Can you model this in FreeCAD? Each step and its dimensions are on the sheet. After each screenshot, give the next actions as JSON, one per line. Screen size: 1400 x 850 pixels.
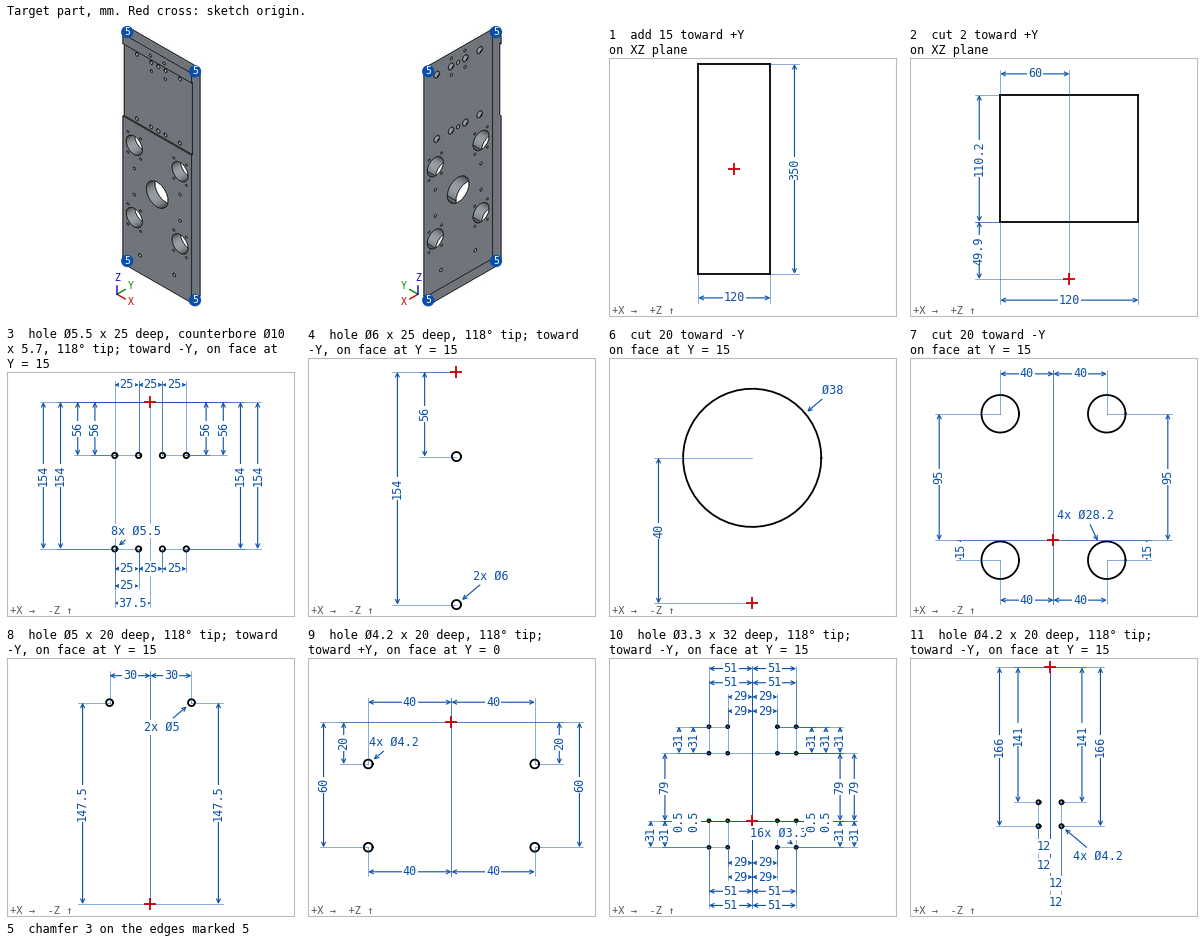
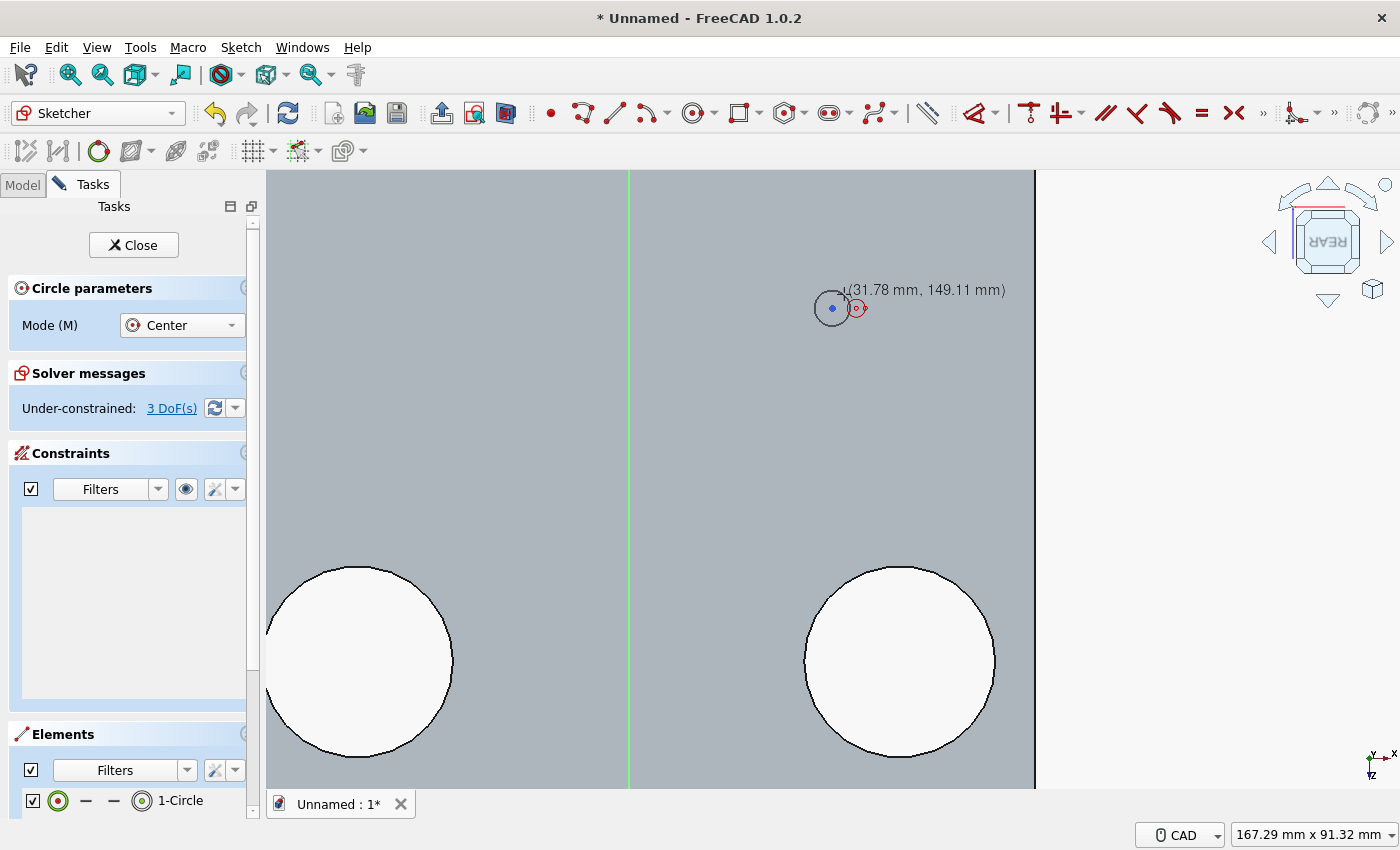
{"action": "scroll", "coordinate": [425, 306], "scroll_direction": "up", "scroll_amount": 2}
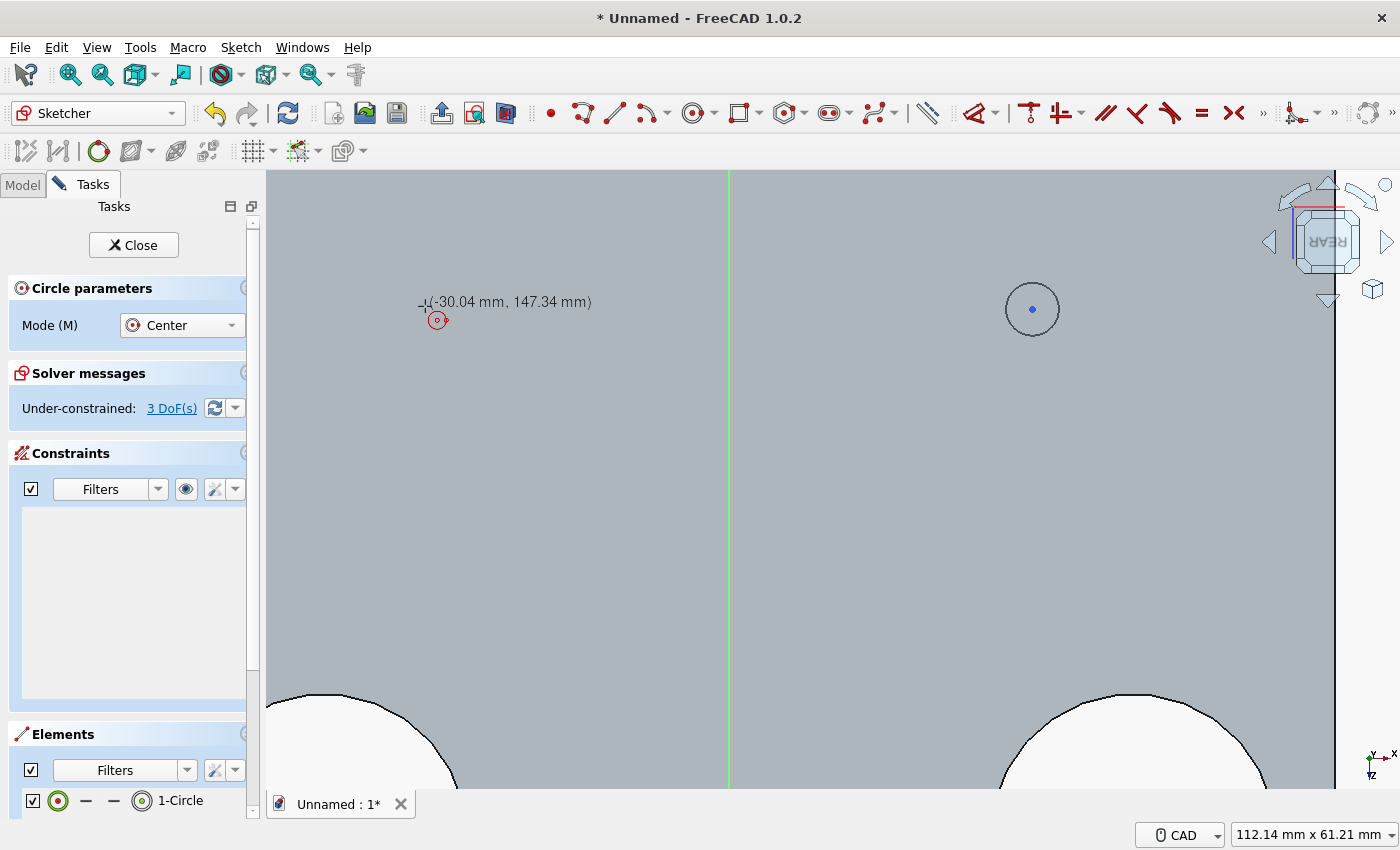
{"action": "scroll", "coordinate": [776, 296], "scroll_direction": "down", "scroll_amount": 7}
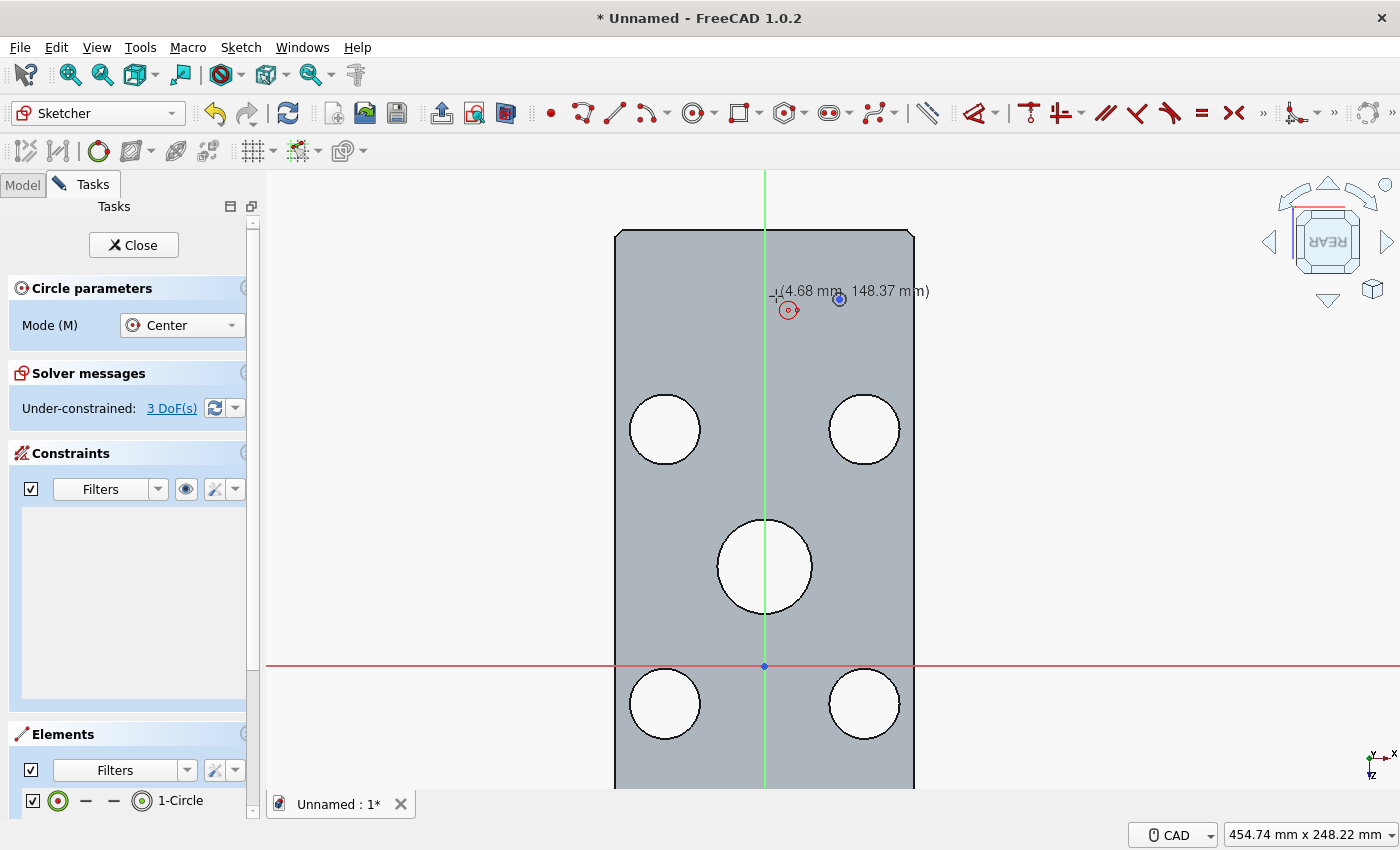
{"action": "left_click", "coordinate": [690, 299]}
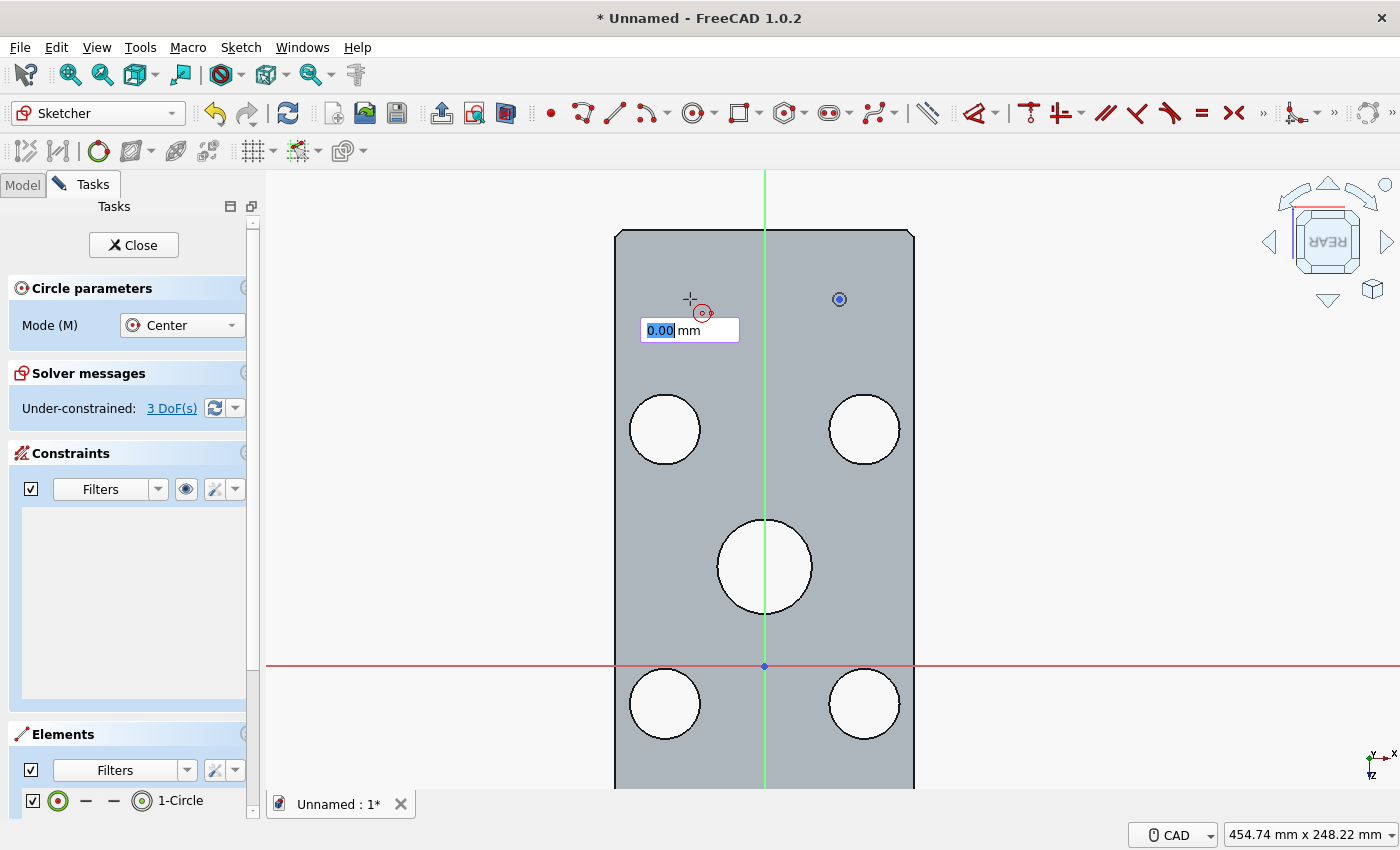
{"action": "scroll", "coordinate": [694, 294], "scroll_direction": "up", "scroll_amount": 5}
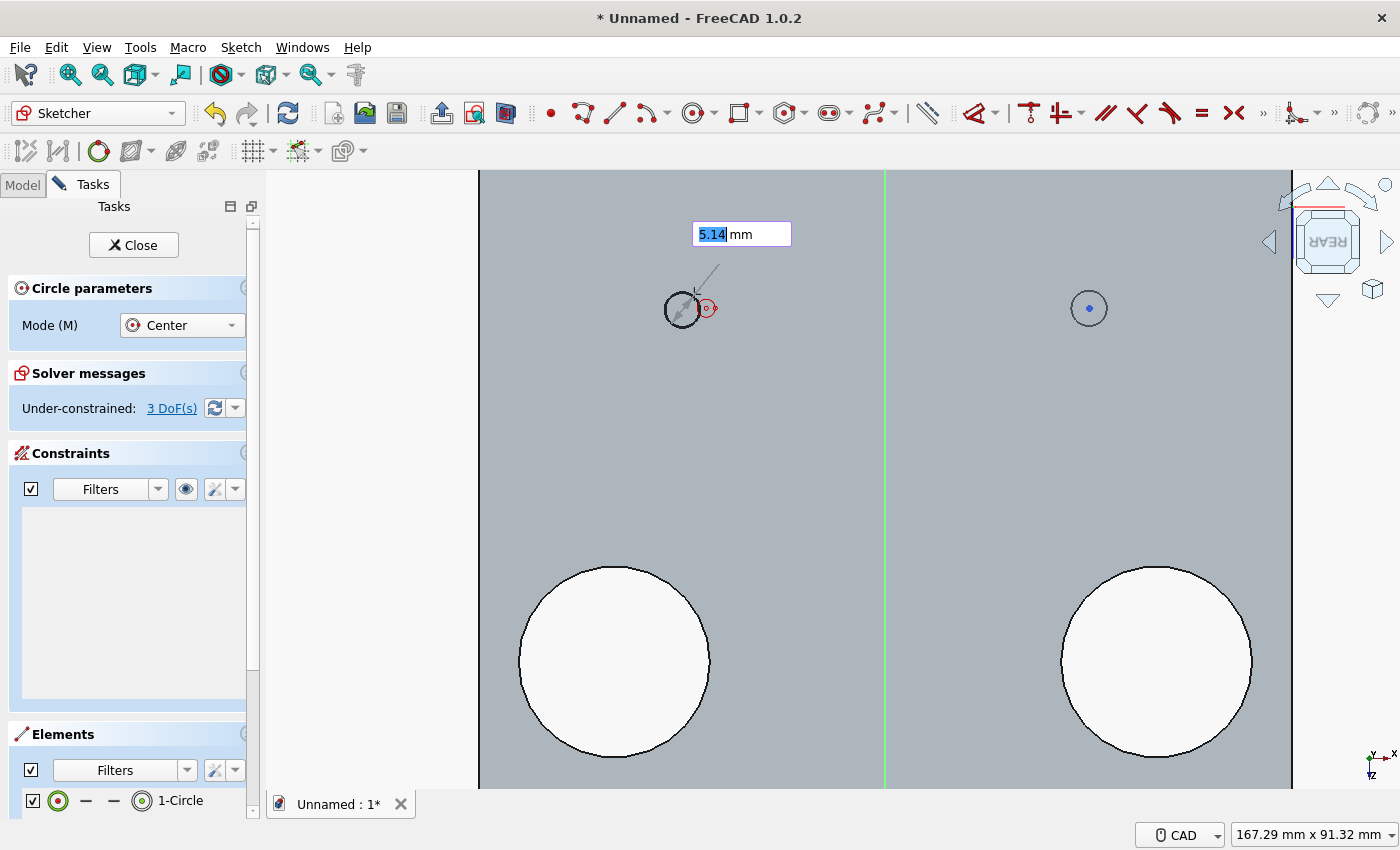
{"action": "left_click", "coordinate": [694, 294]}
{"action": "key", "text": "Escape"}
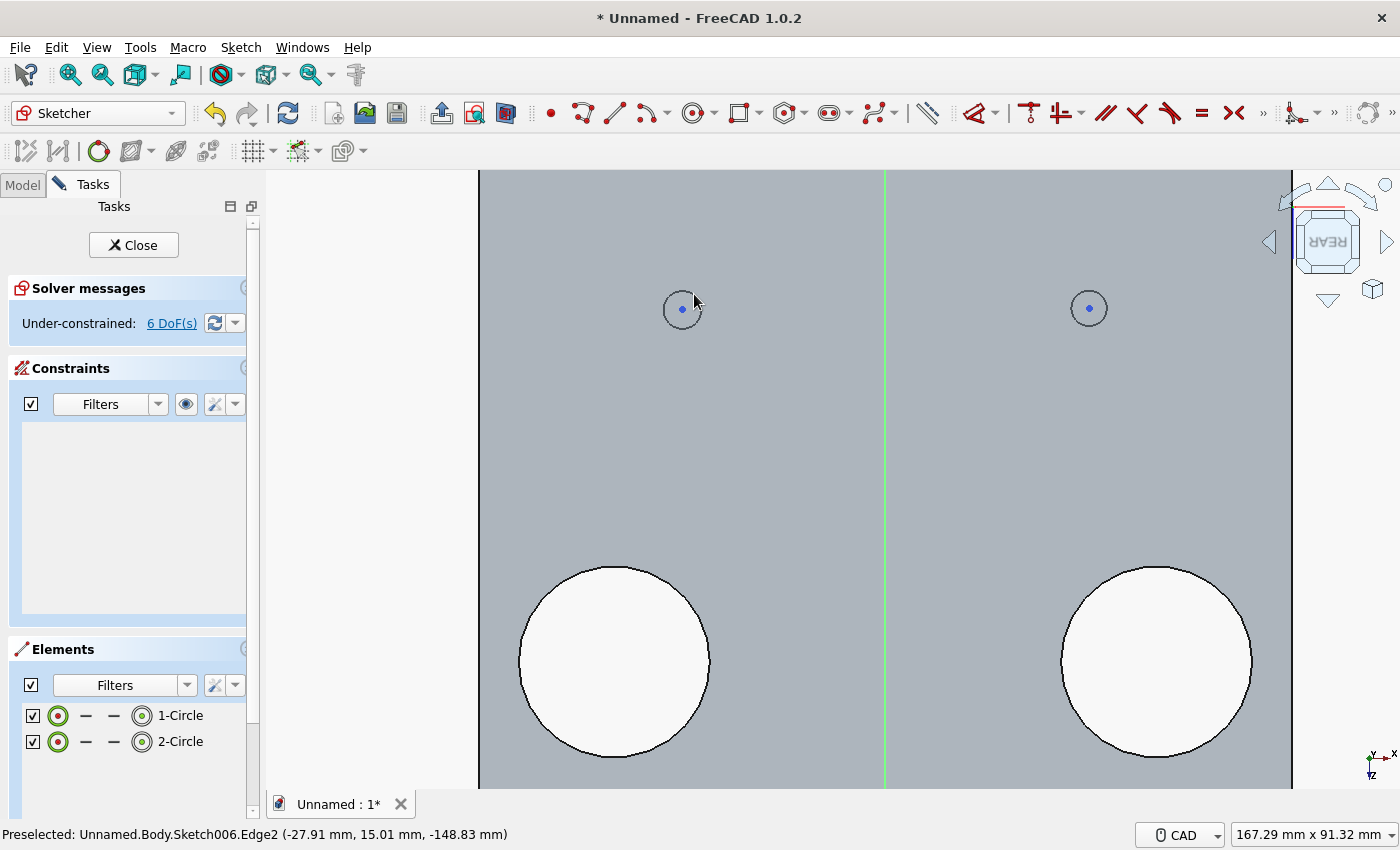
{"action": "left_click", "coordinate": [1102, 296]}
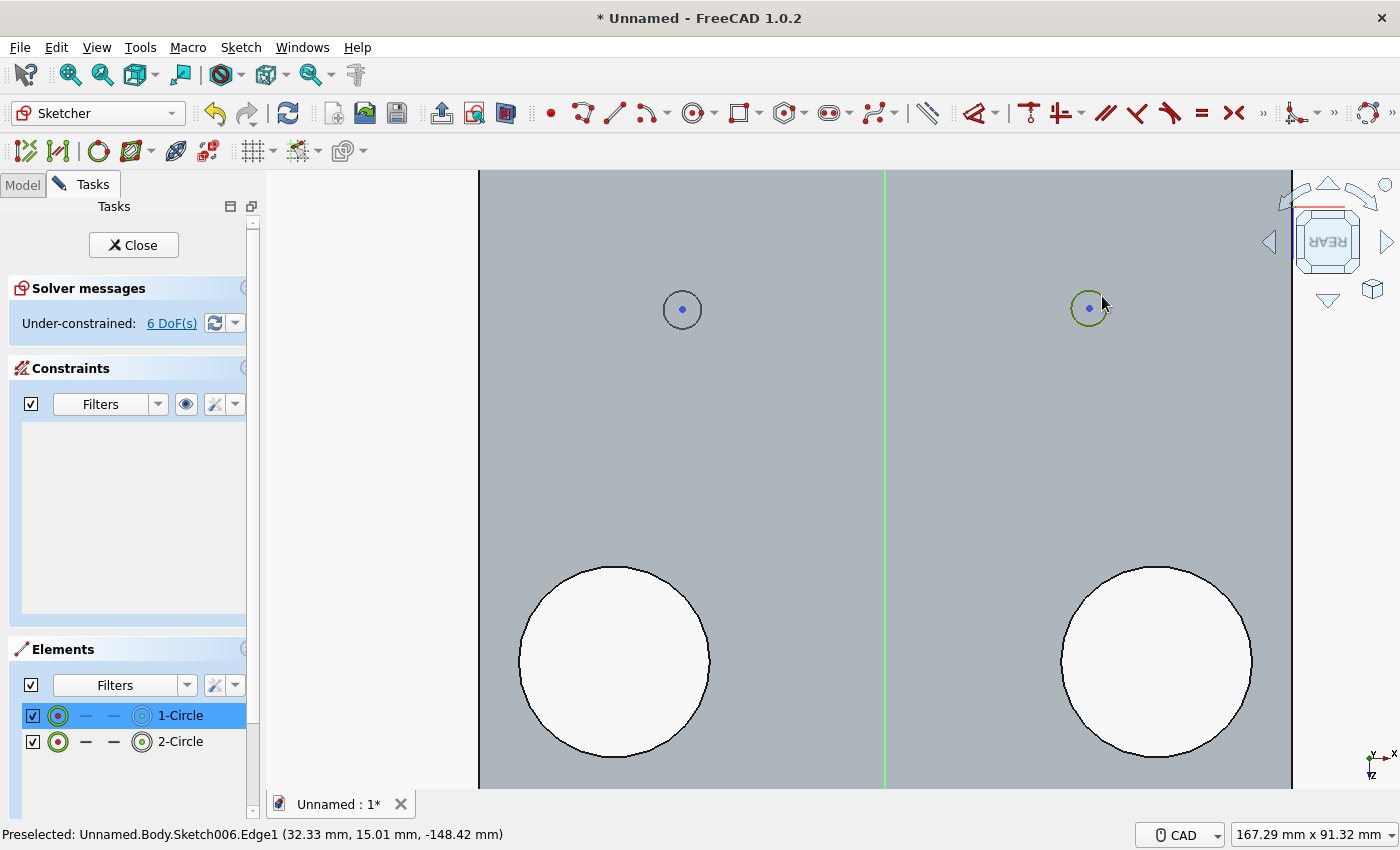
{"action": "left_click", "coordinate": [696, 297]}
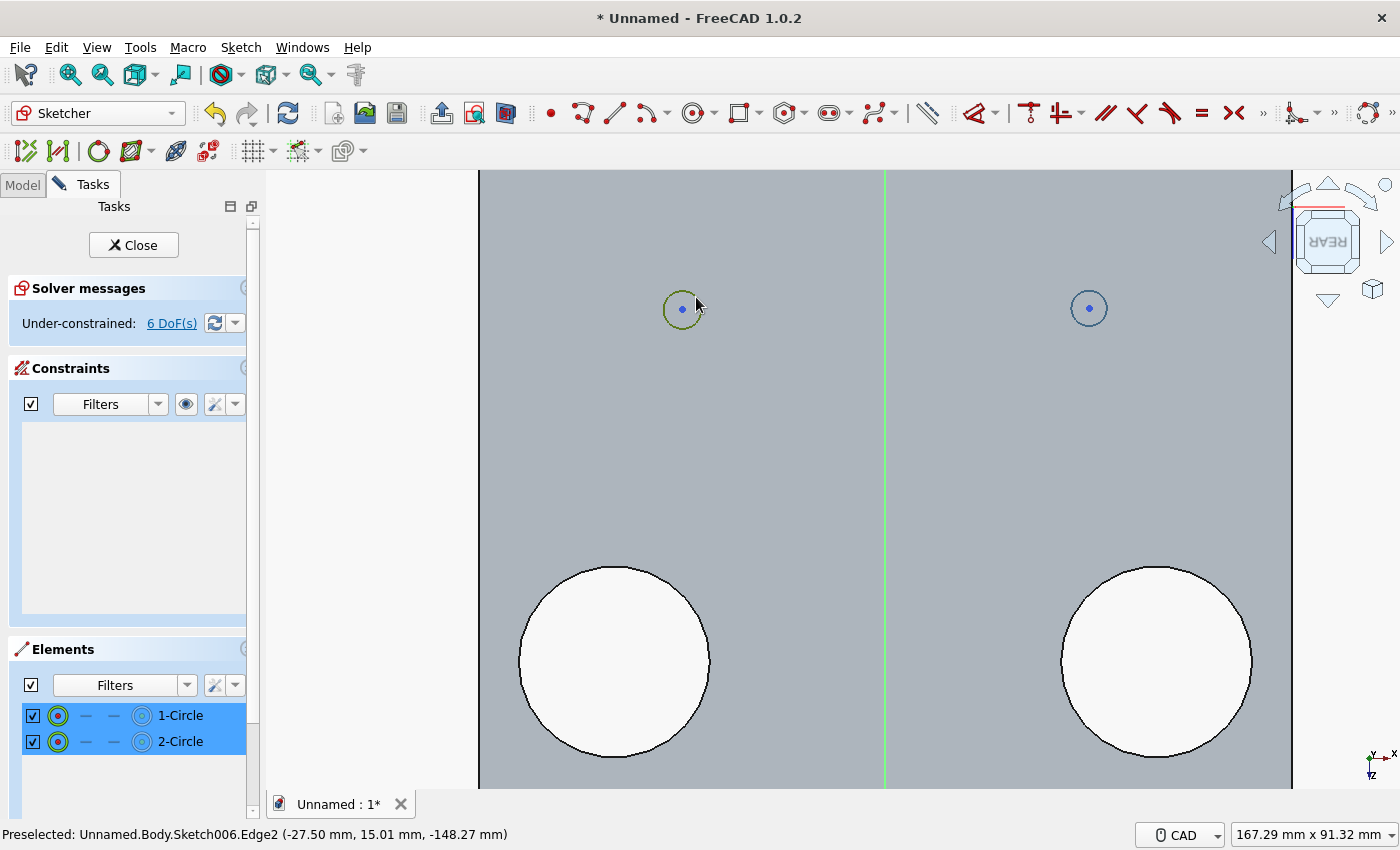
{"action": "left_click", "coordinate": [1202, 114]}